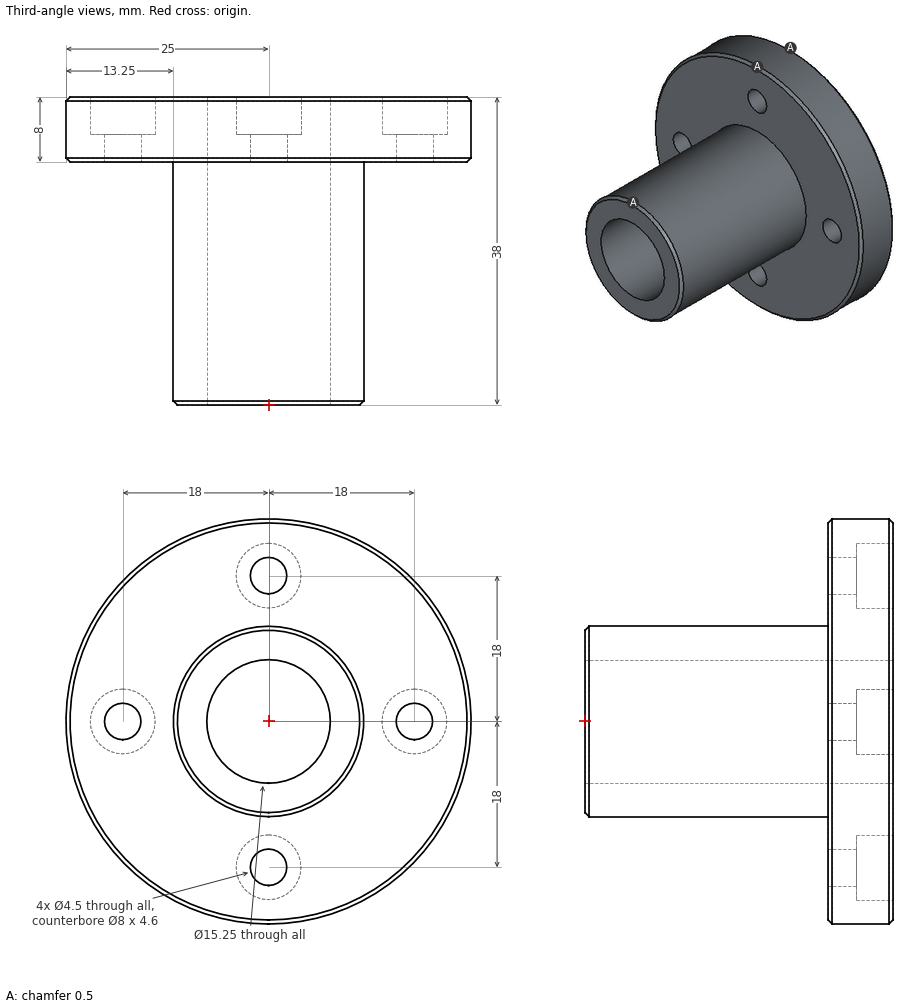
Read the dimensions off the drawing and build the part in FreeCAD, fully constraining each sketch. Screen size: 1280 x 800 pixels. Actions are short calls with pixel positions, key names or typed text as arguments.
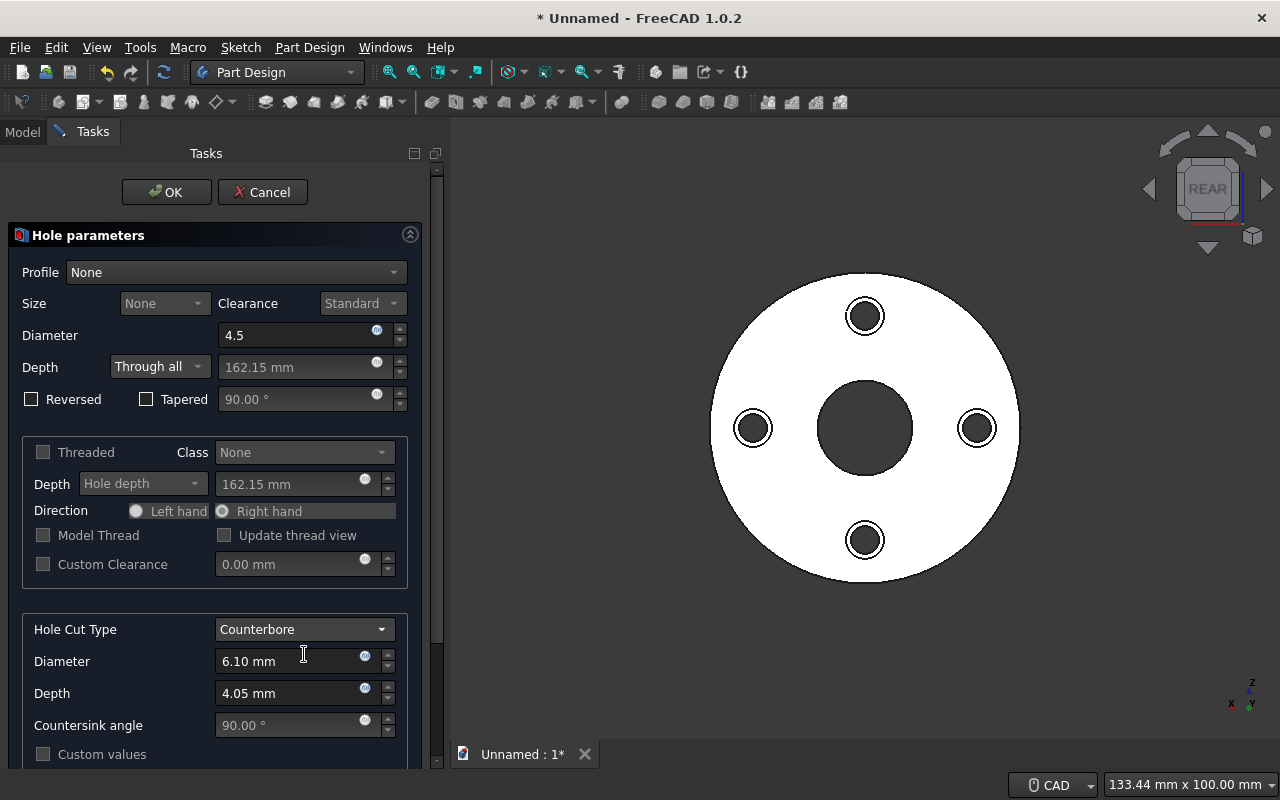
triple_click(298, 661)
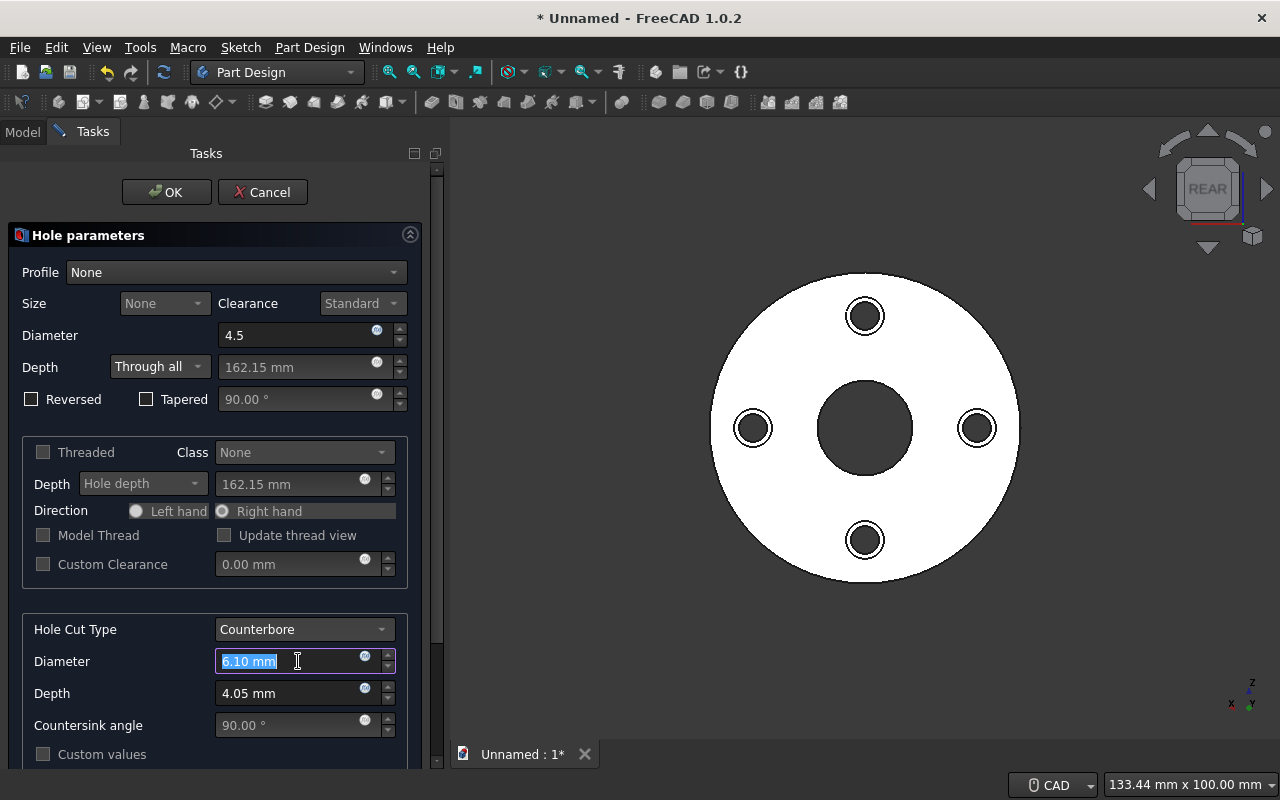
text(8)
key(Tab)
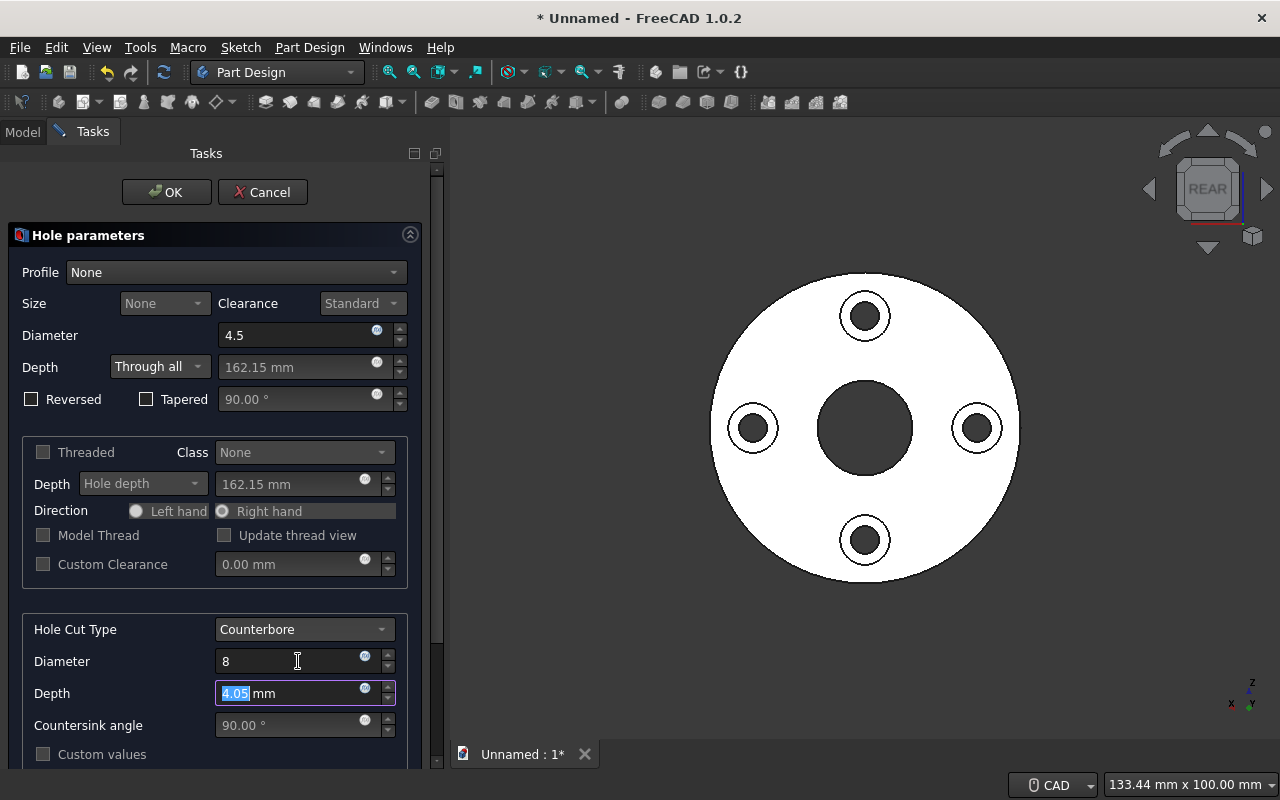
text(4.6)
key(Tab)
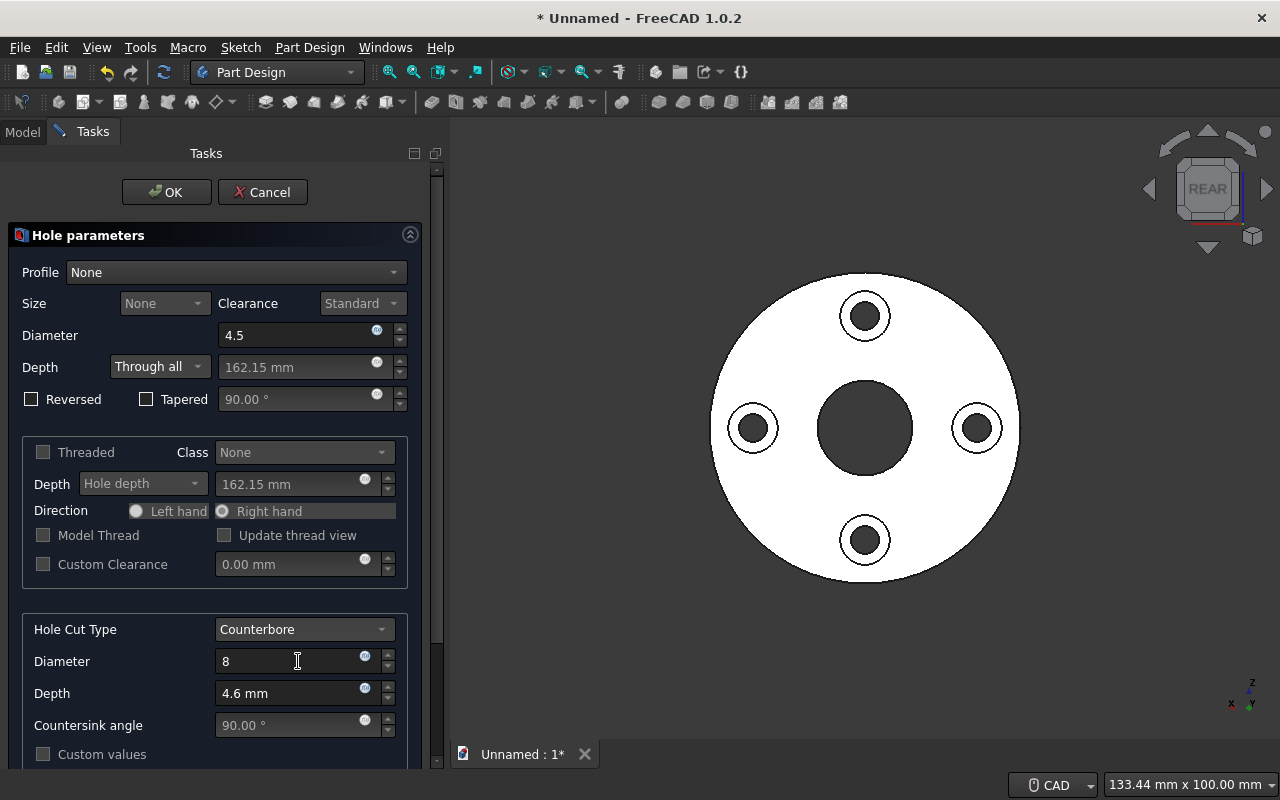
click(167, 192)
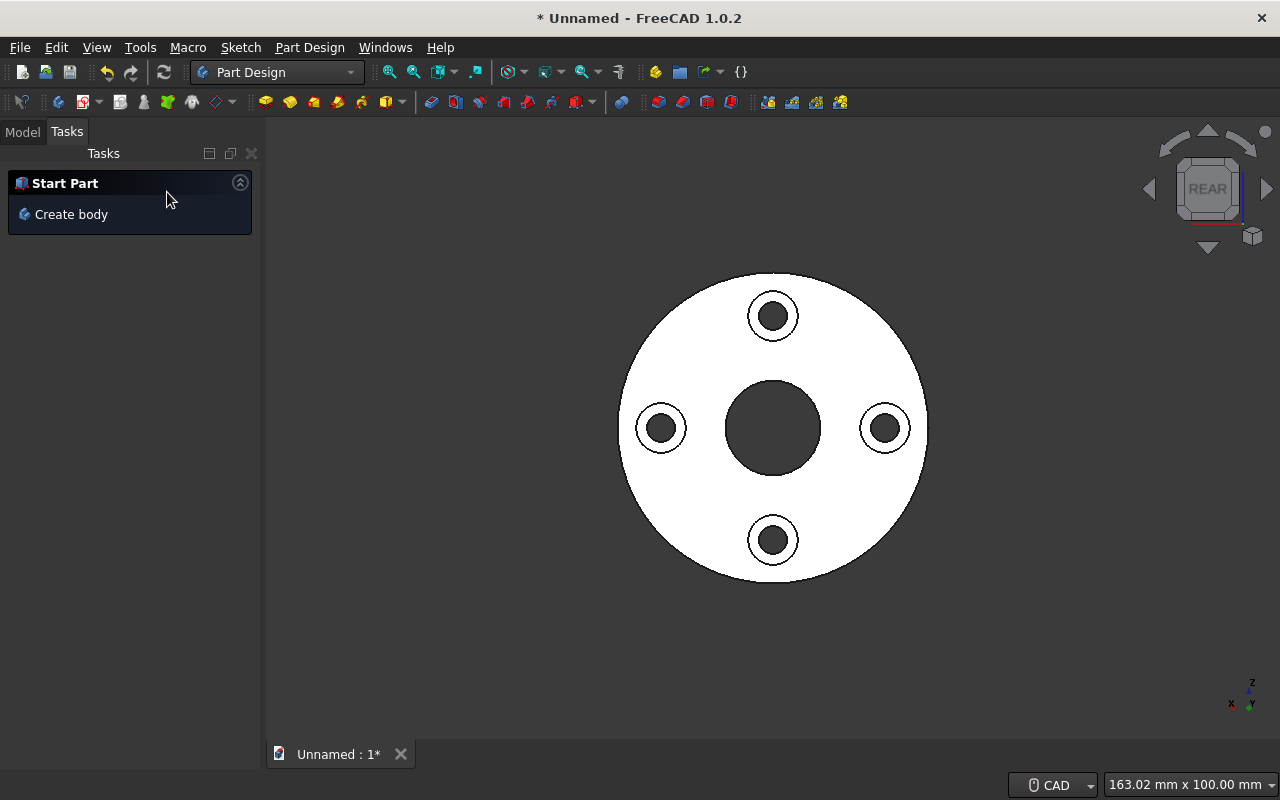
click(821, 279)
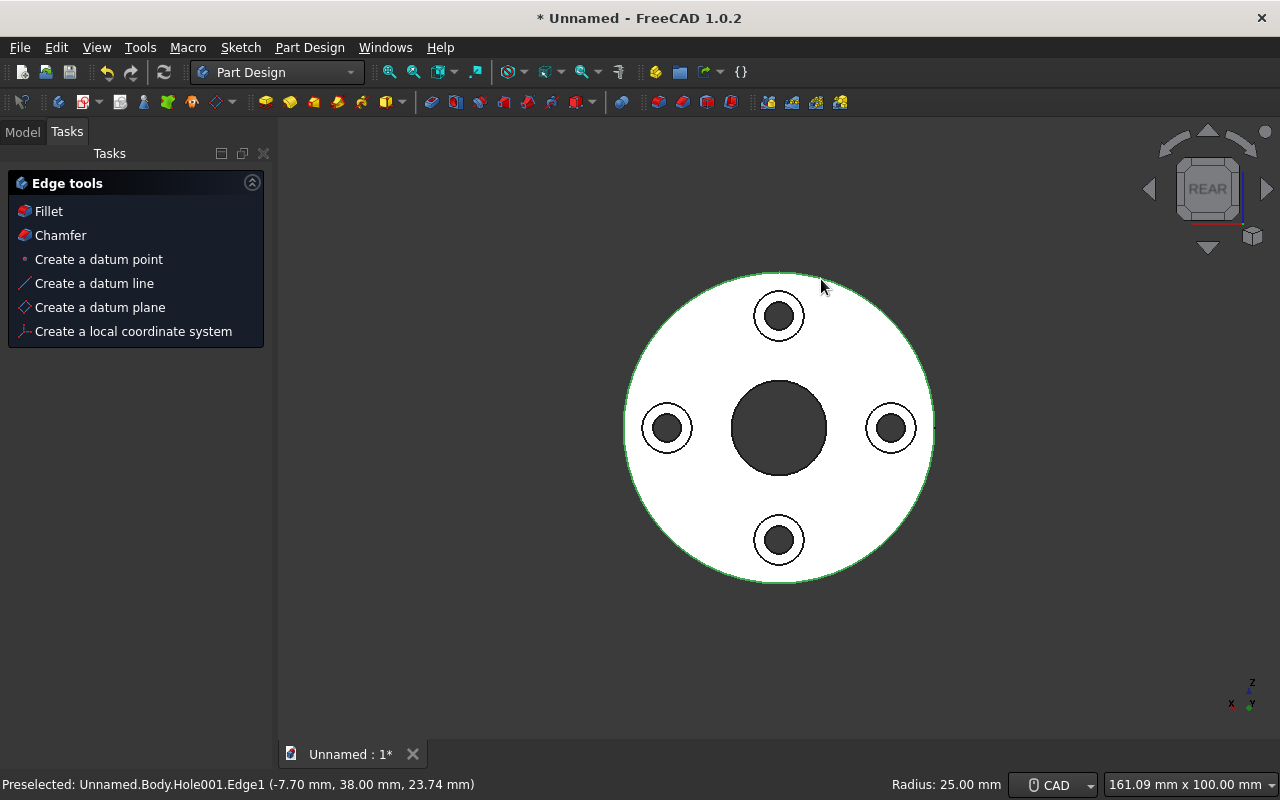
key(0)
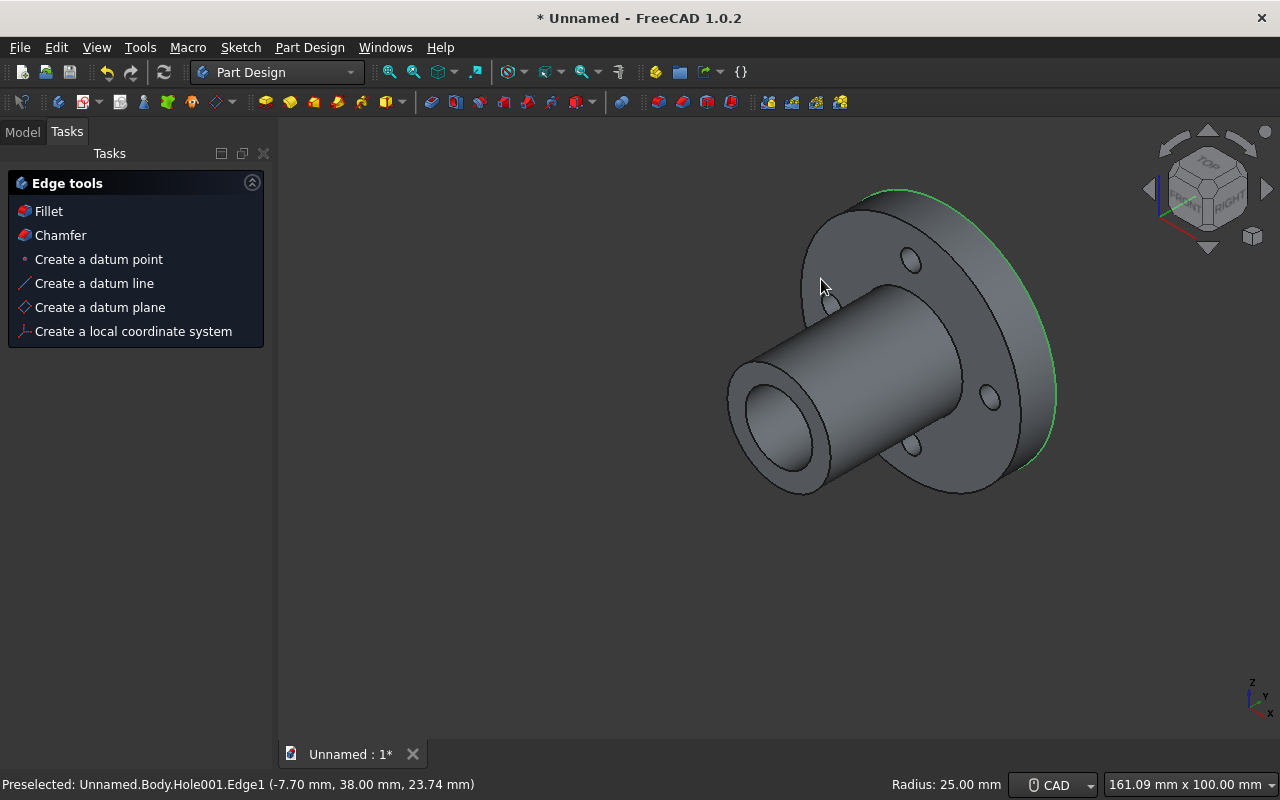
click(831, 457, ctrl)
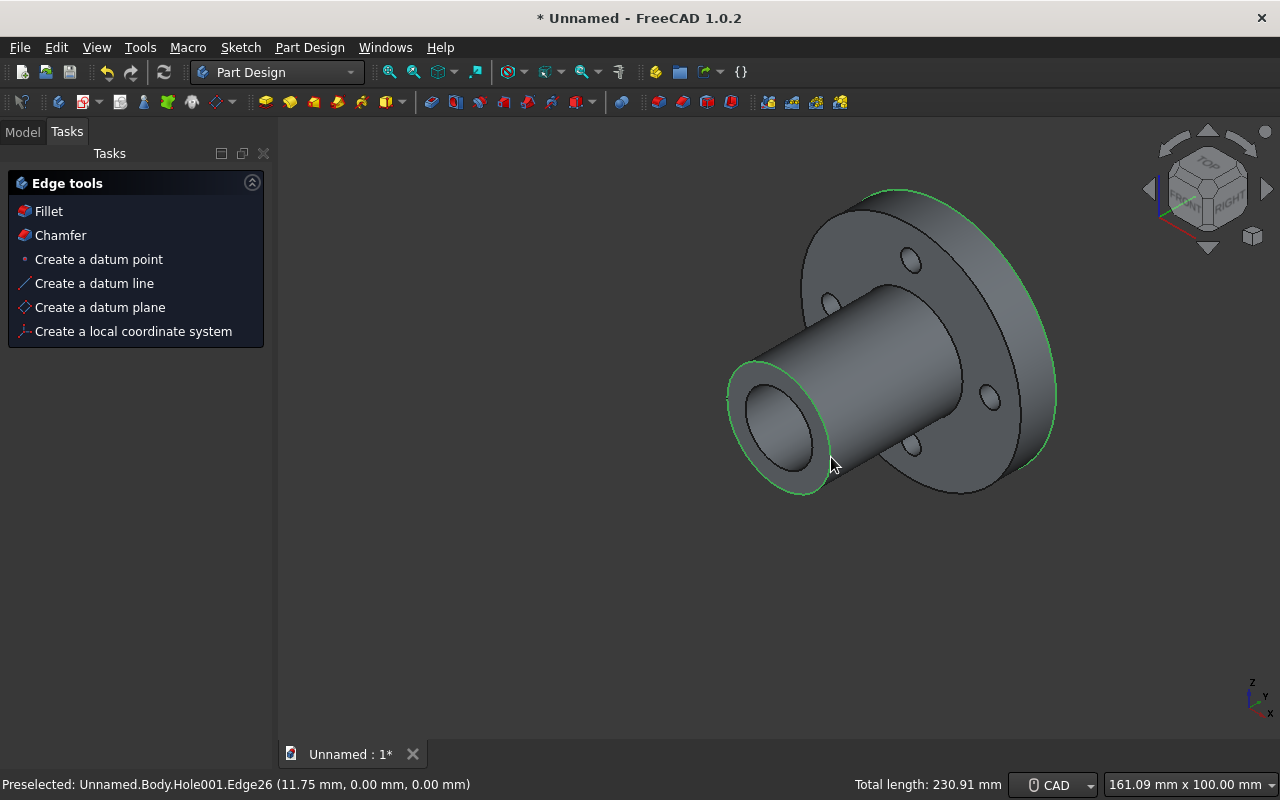
click(1021, 414, ctrl)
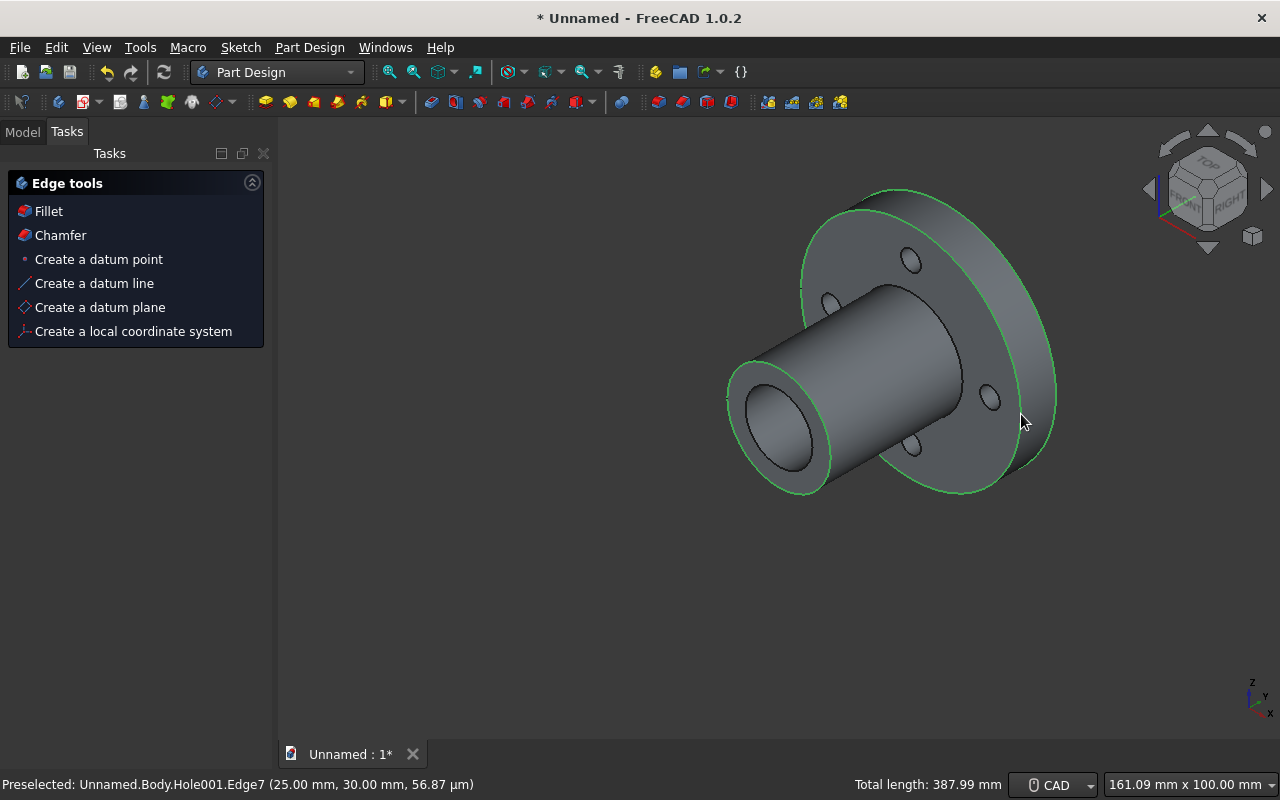
click(684, 102)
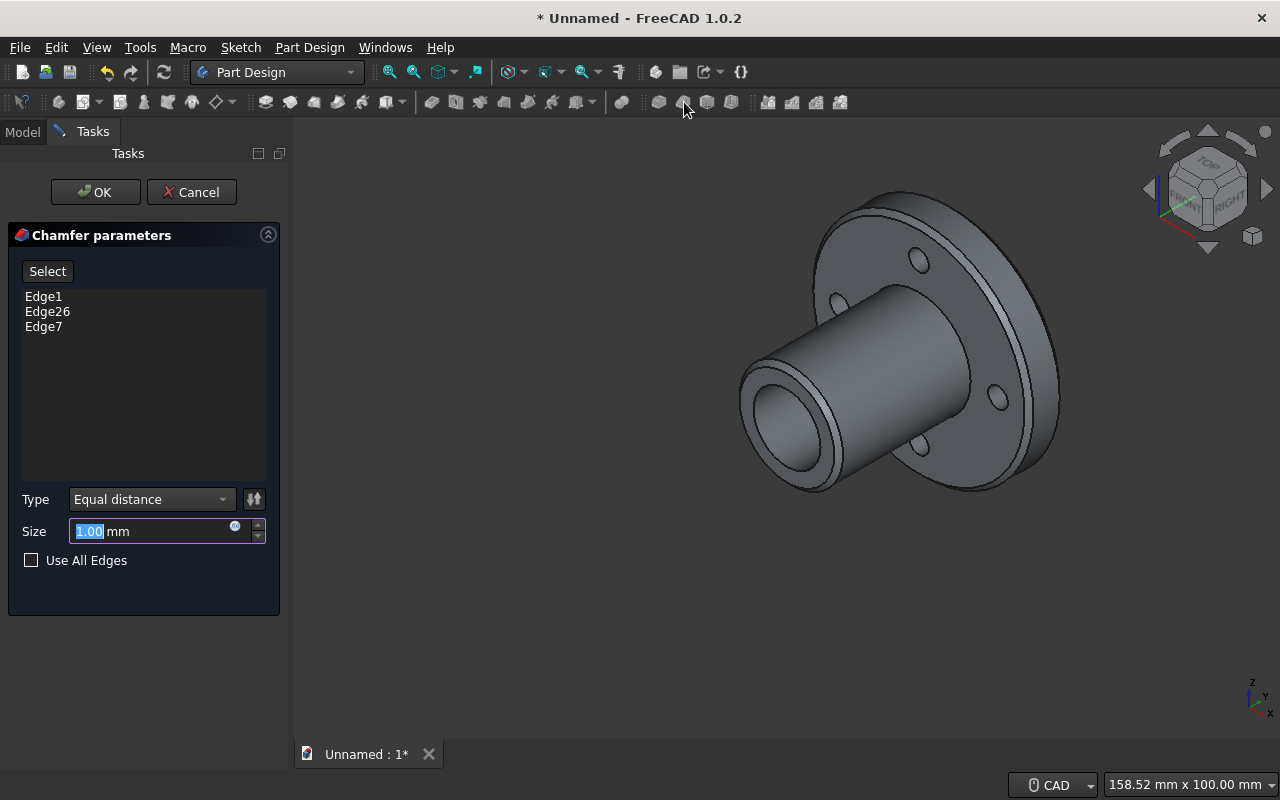
text(0.5)
key(Tab)